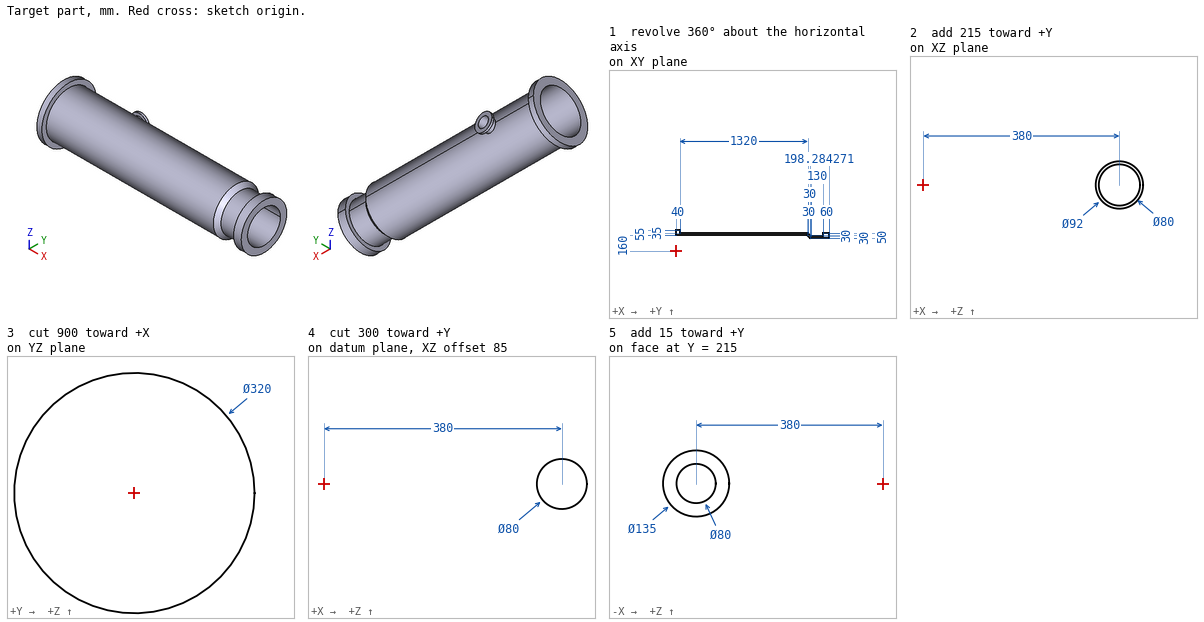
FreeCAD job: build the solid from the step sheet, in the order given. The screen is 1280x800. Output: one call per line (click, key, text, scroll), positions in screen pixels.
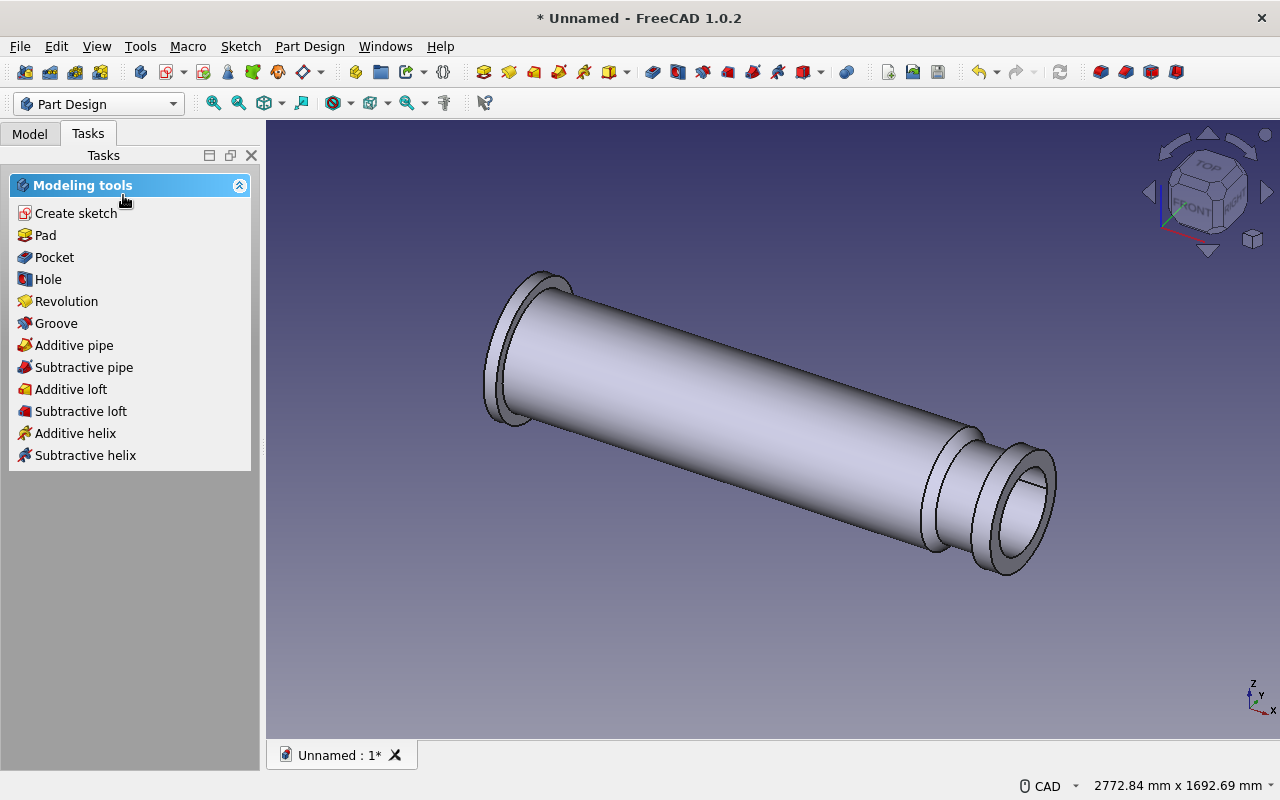
click(653, 72)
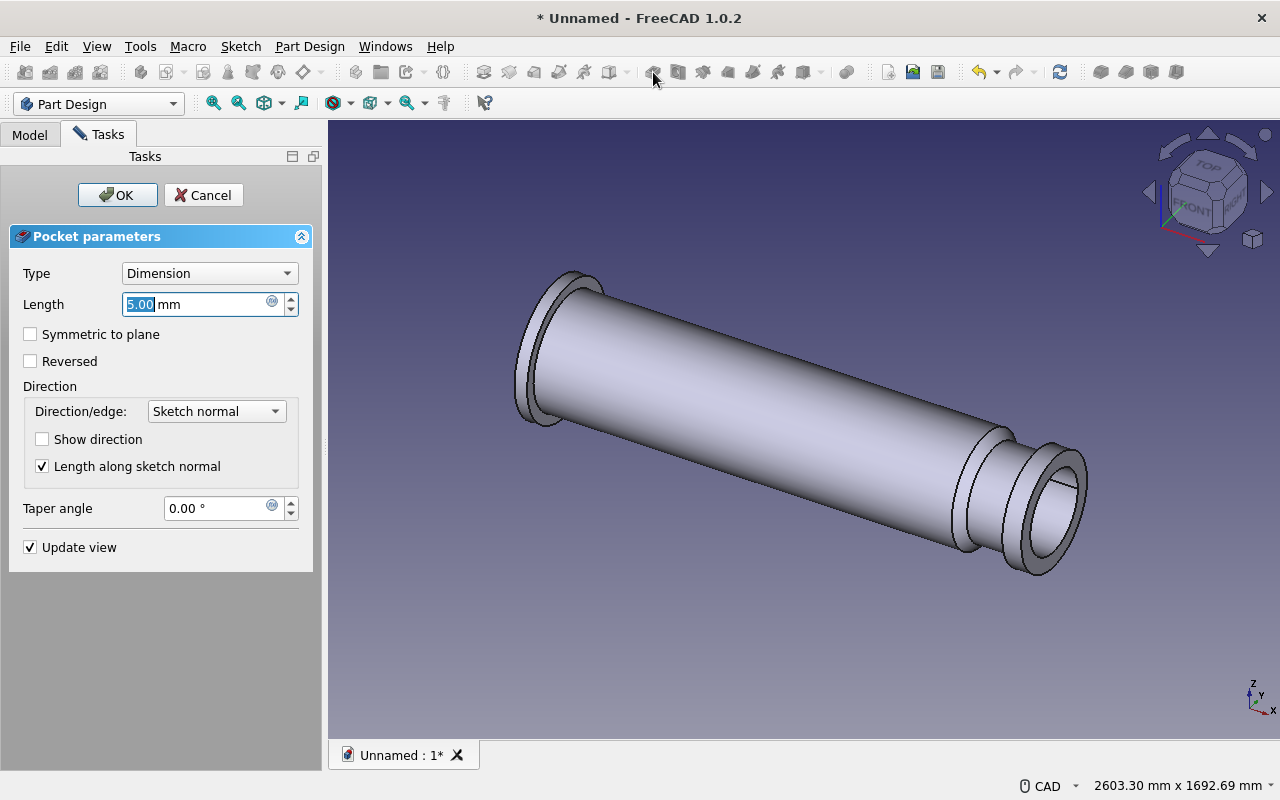
text(900)
key(Tab)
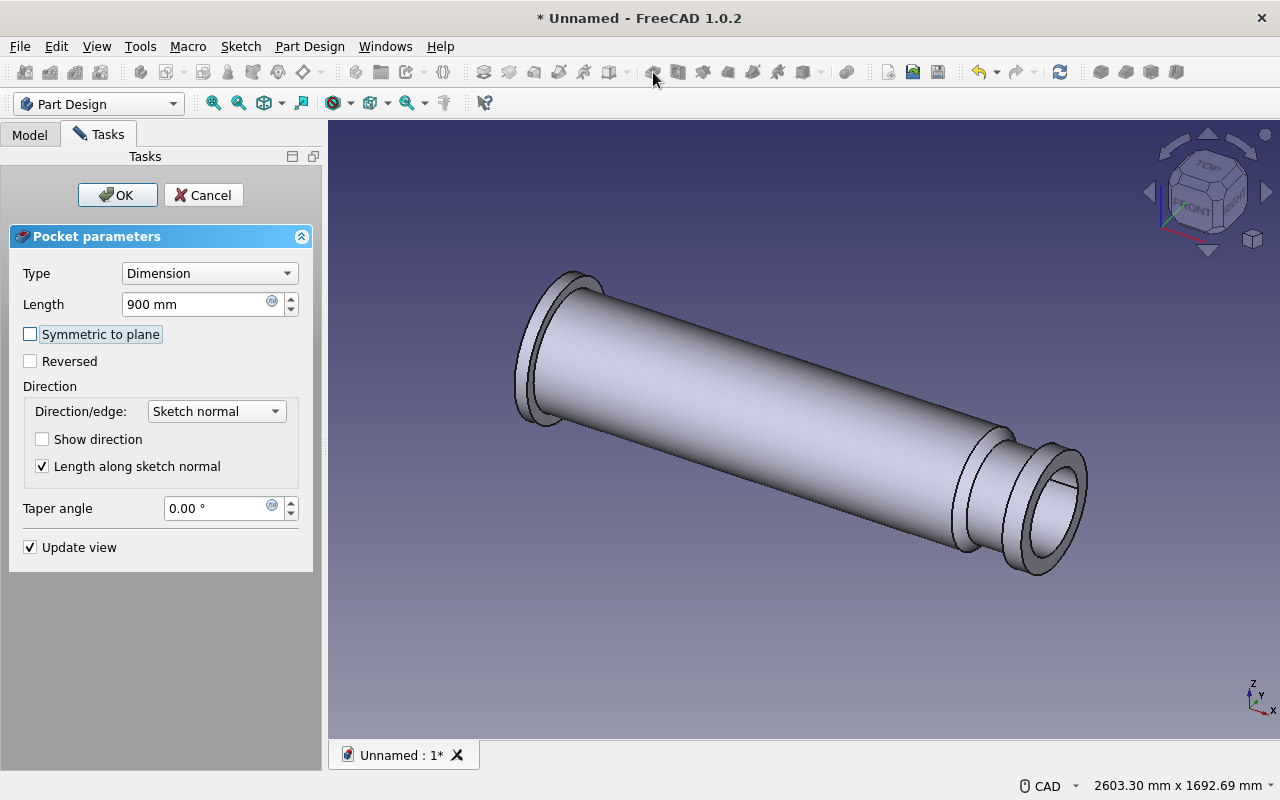
click(31, 361)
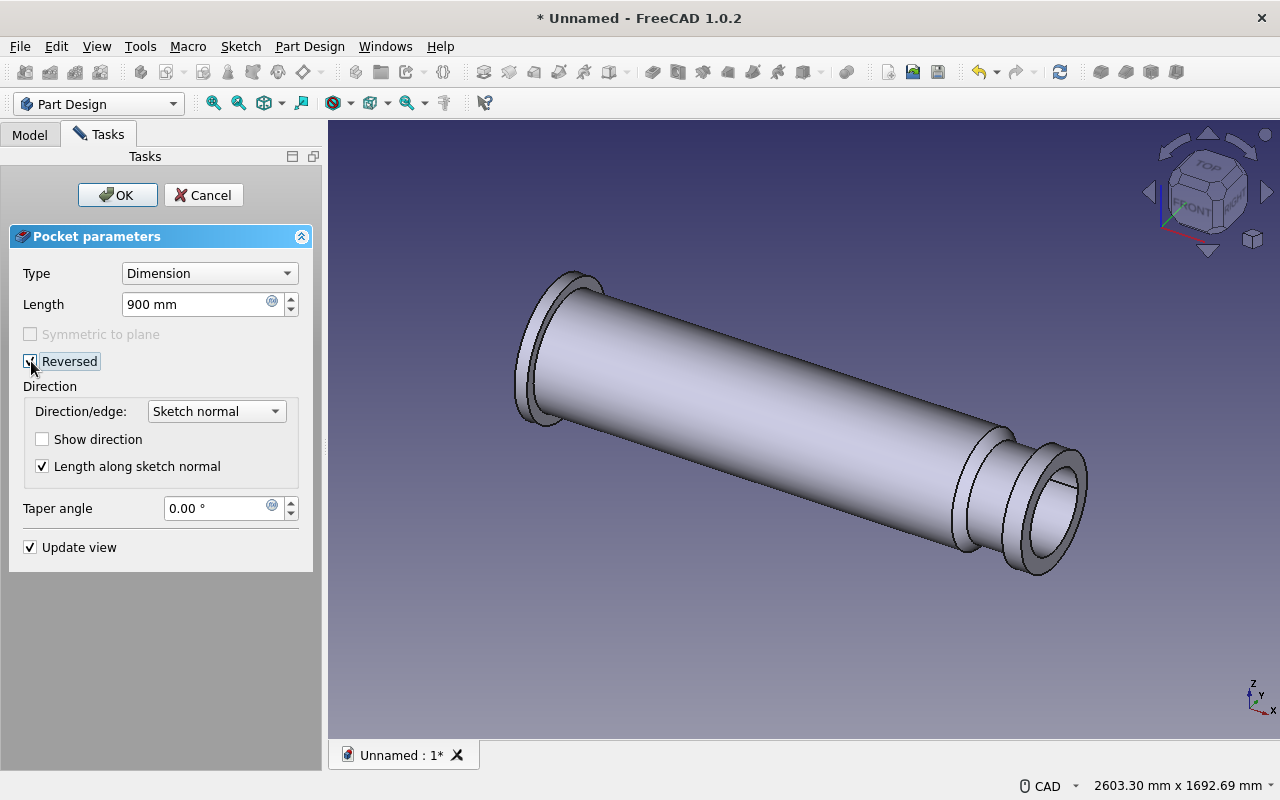
click(118, 195)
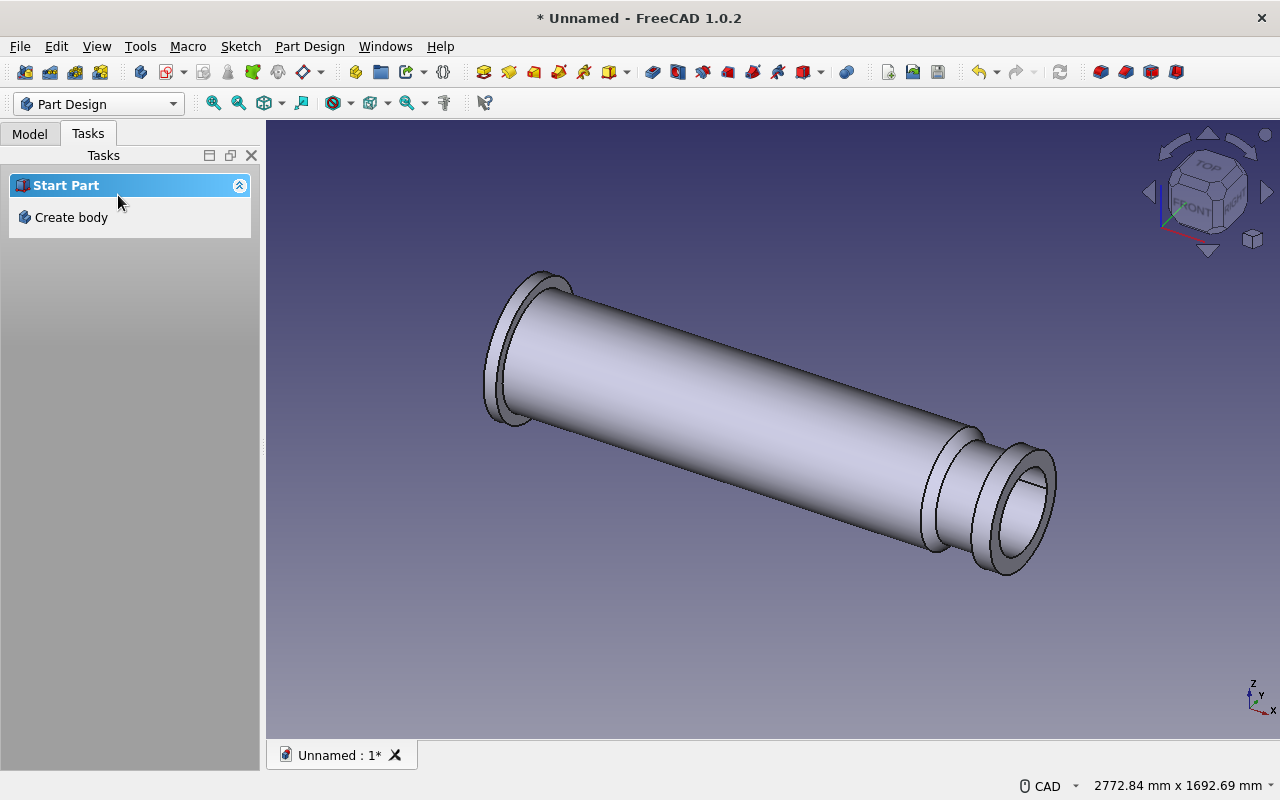
click(30, 134)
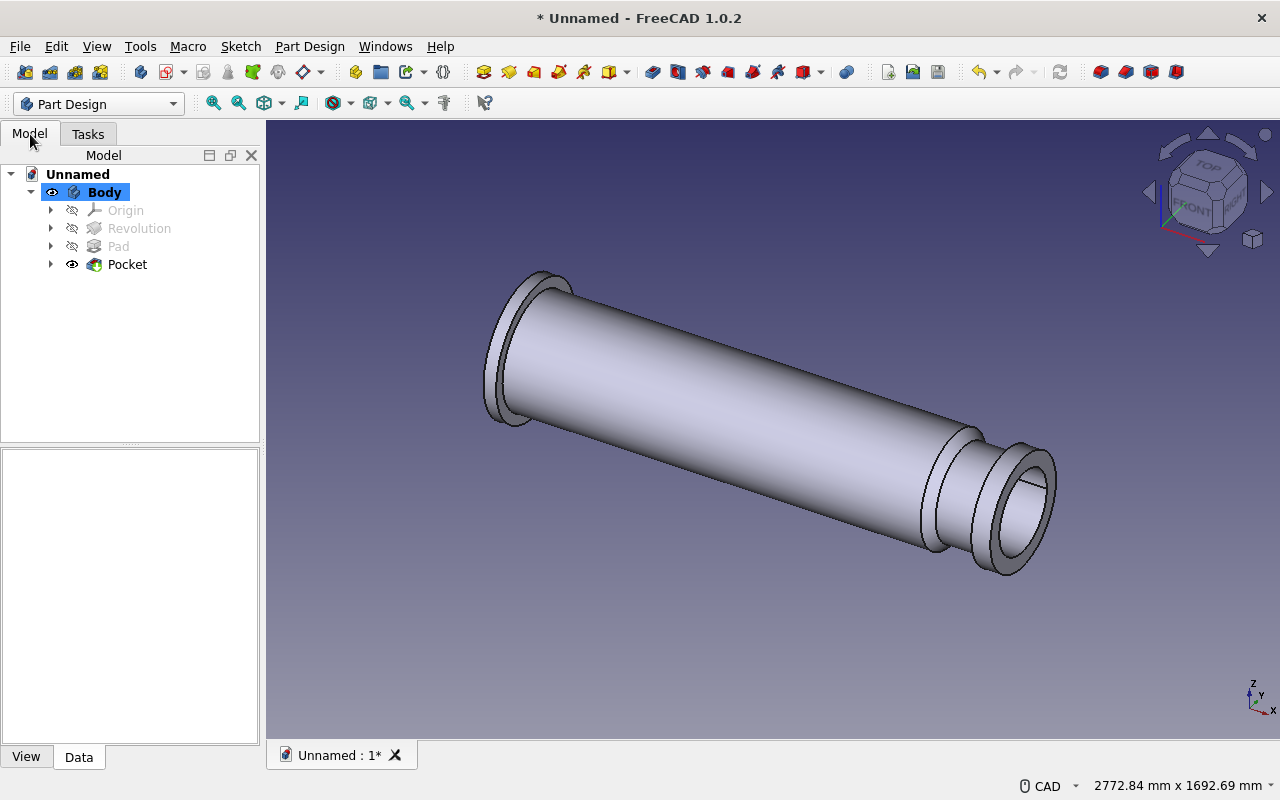
click(51, 210)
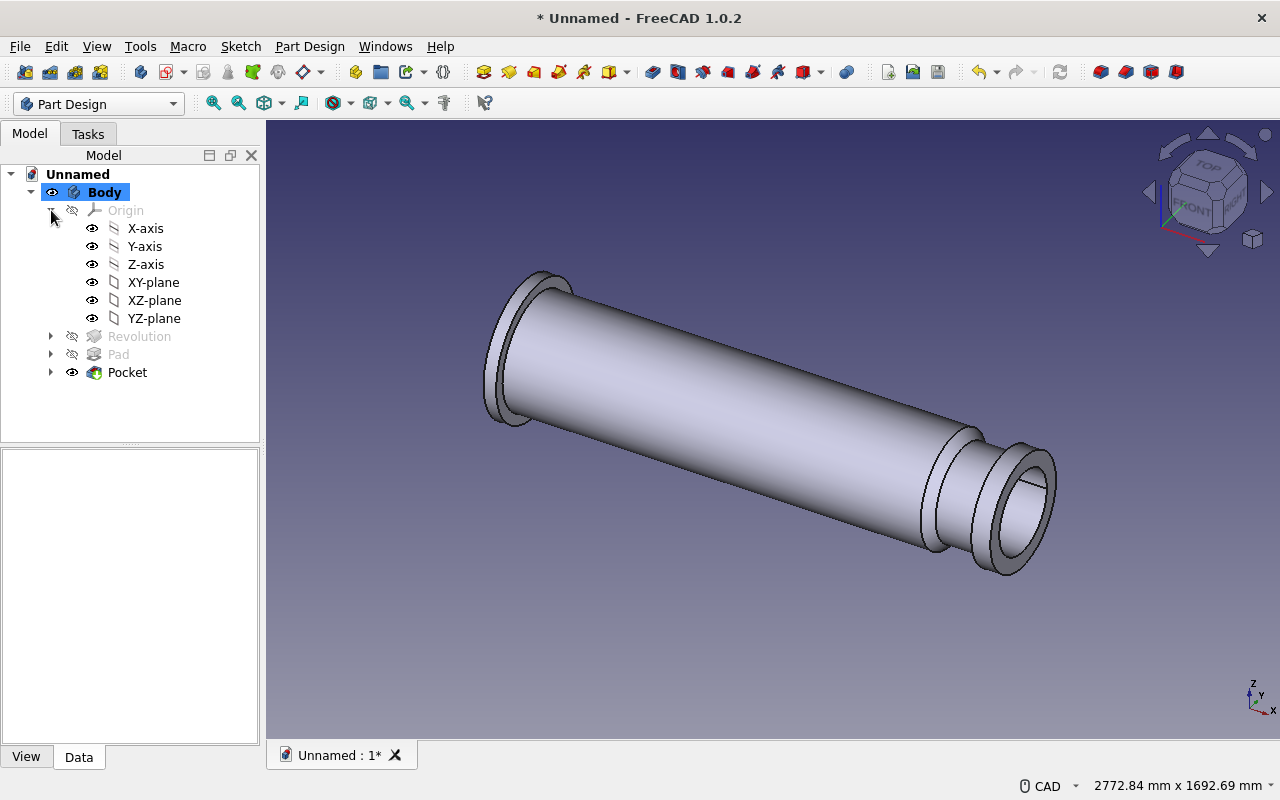
click(137, 300)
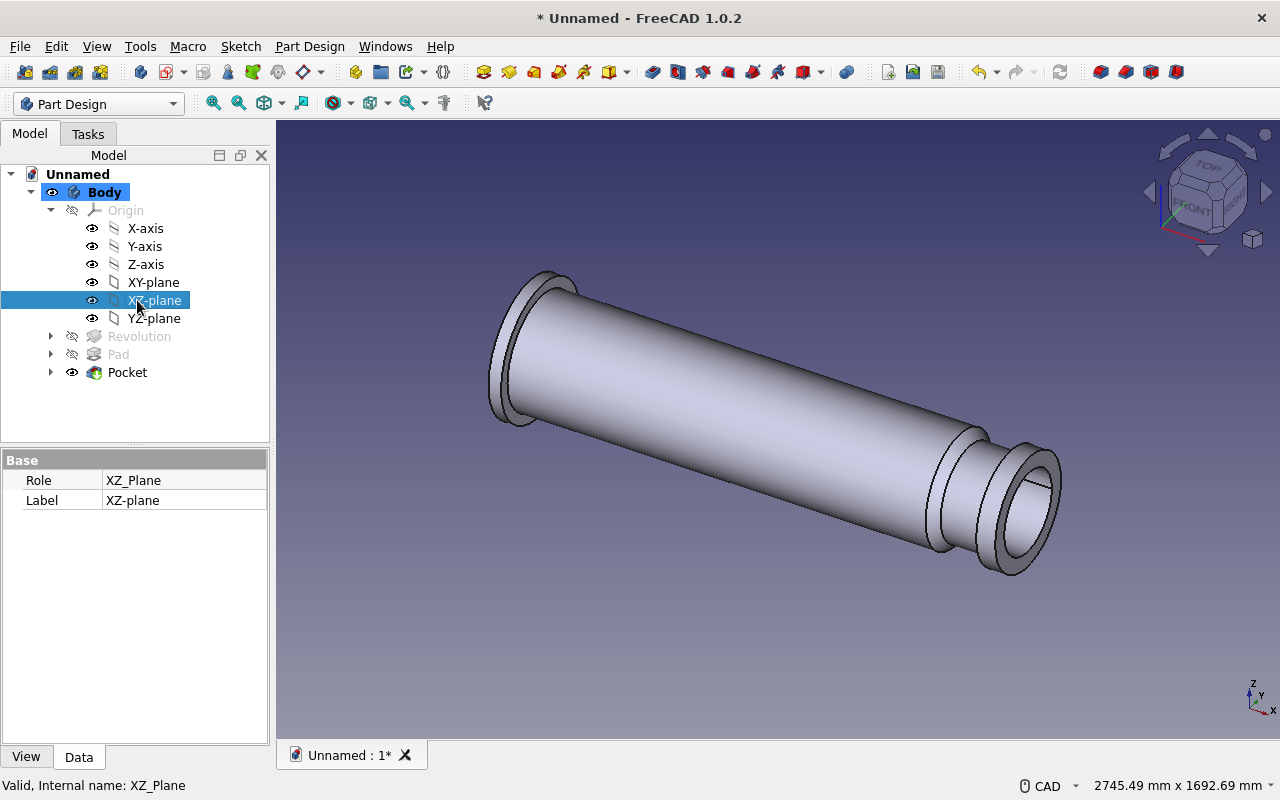
click(302, 72)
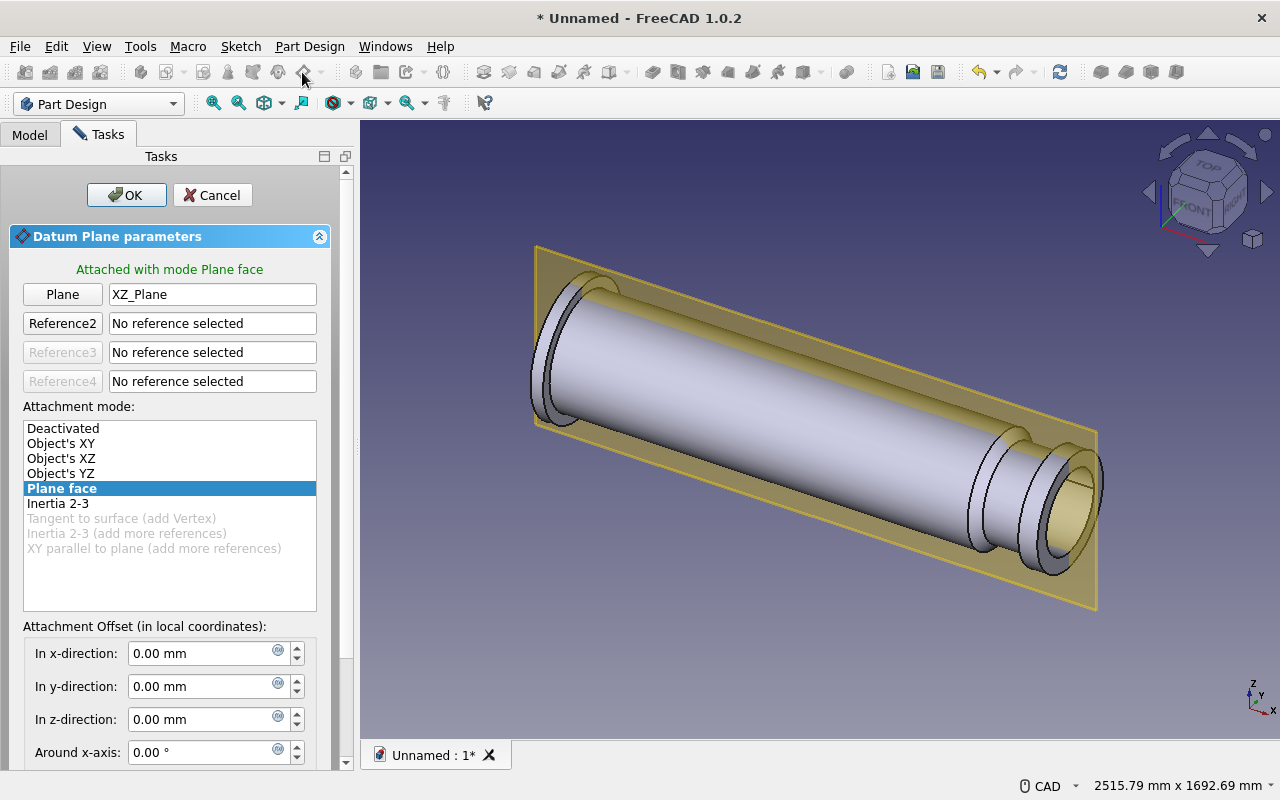
triple_click(210, 720)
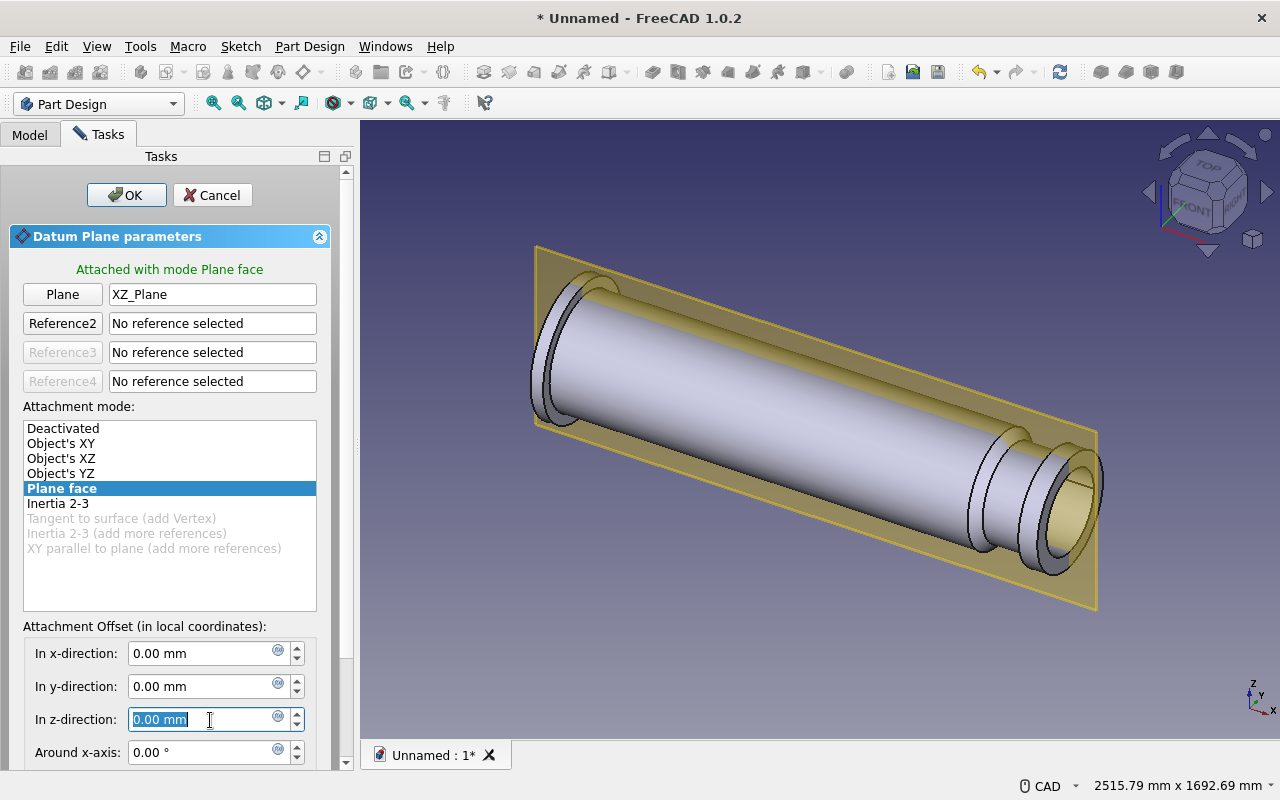
text(85)
key(Tab)